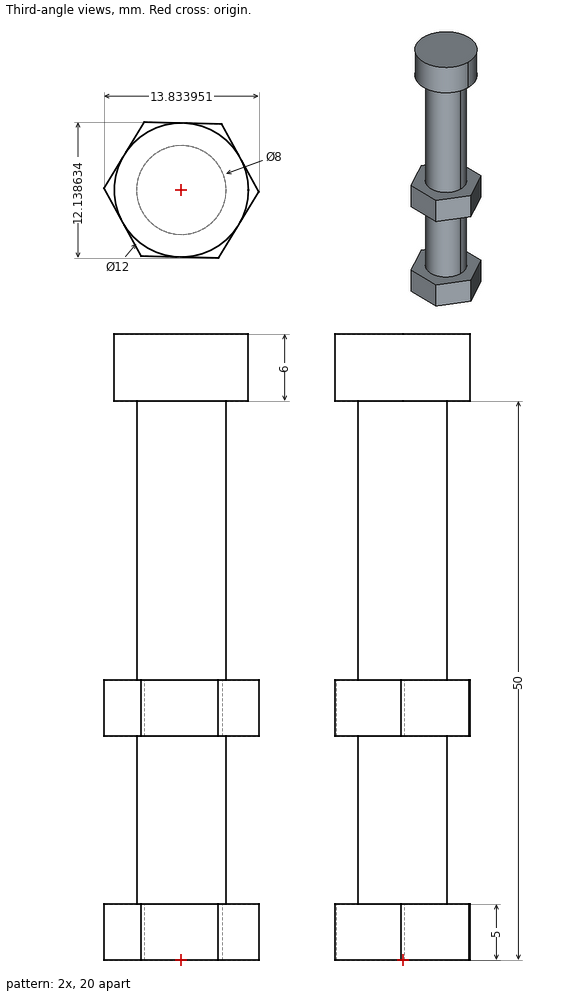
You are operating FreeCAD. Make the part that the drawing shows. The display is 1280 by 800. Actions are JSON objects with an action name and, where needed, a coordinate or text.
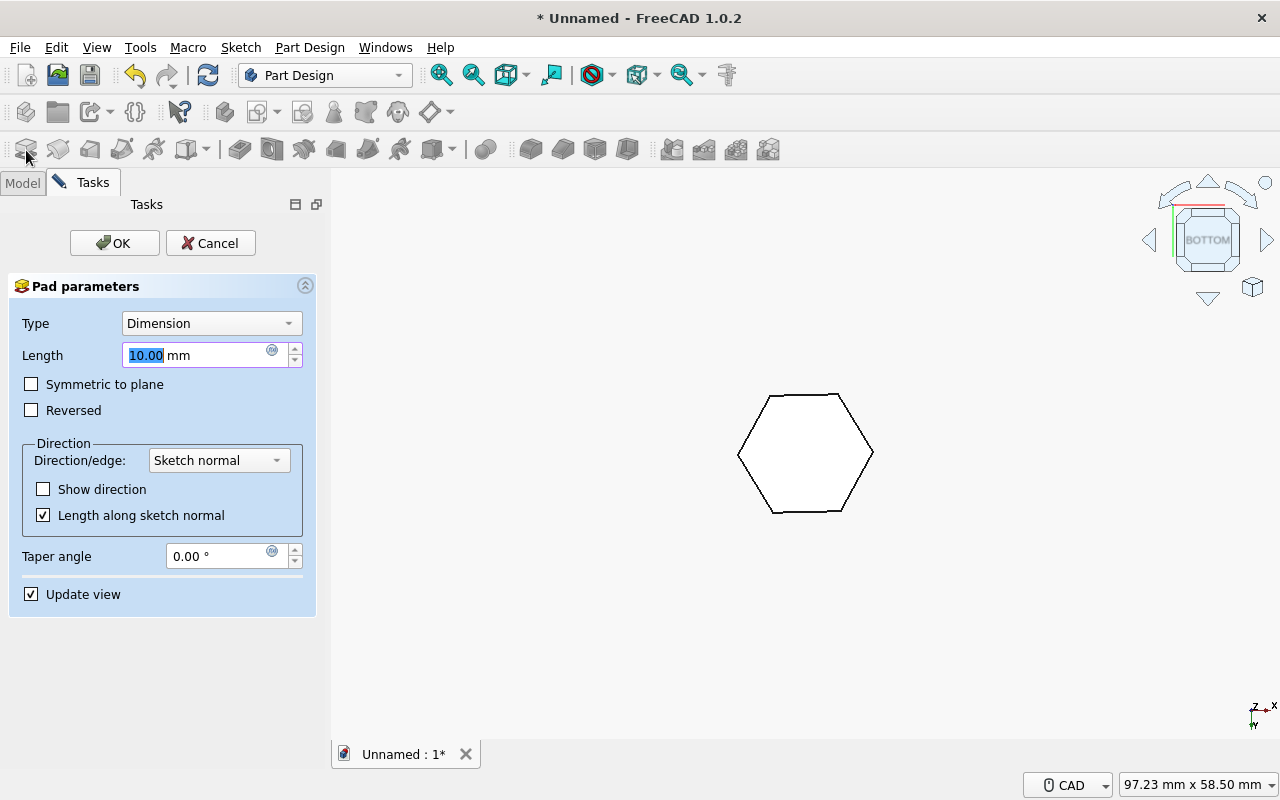
{"action": "type", "text": "5"}
{"action": "key", "text": "Tab"}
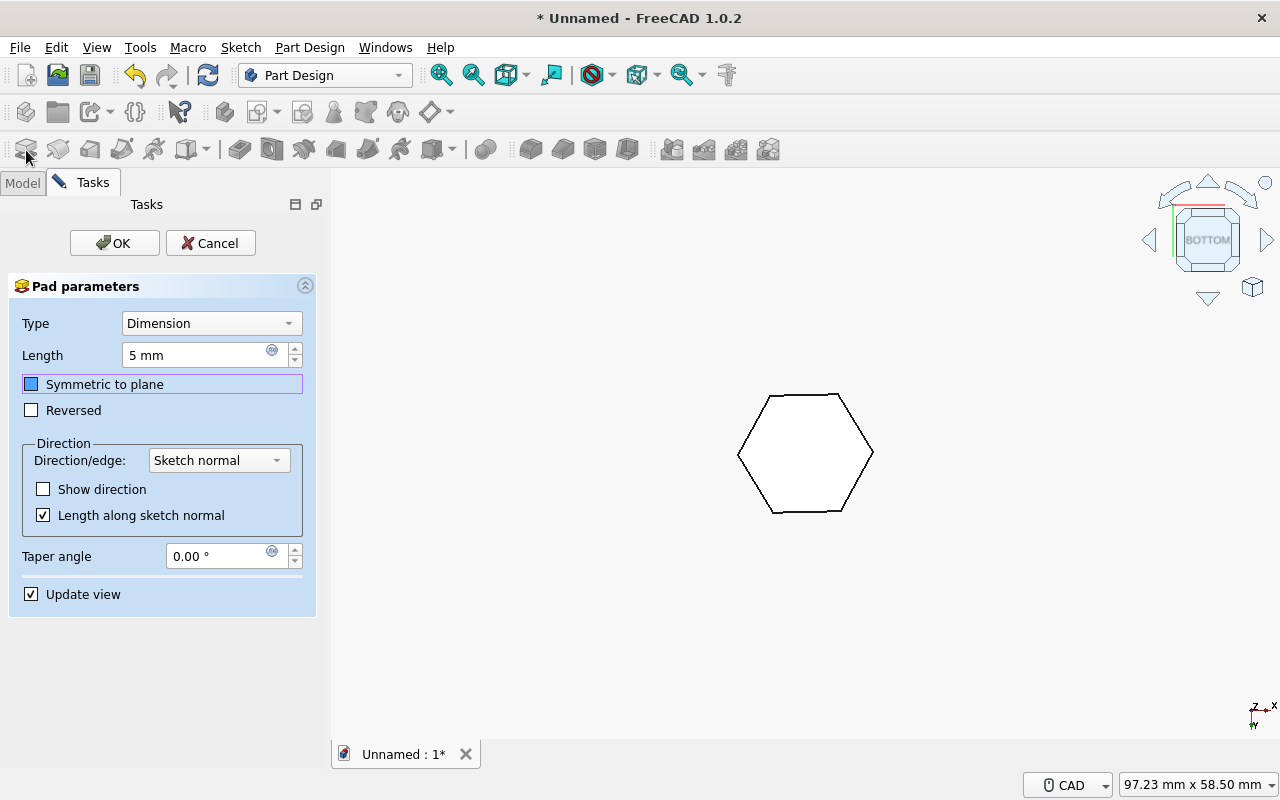
{"action": "left_click", "coordinate": [30, 410]}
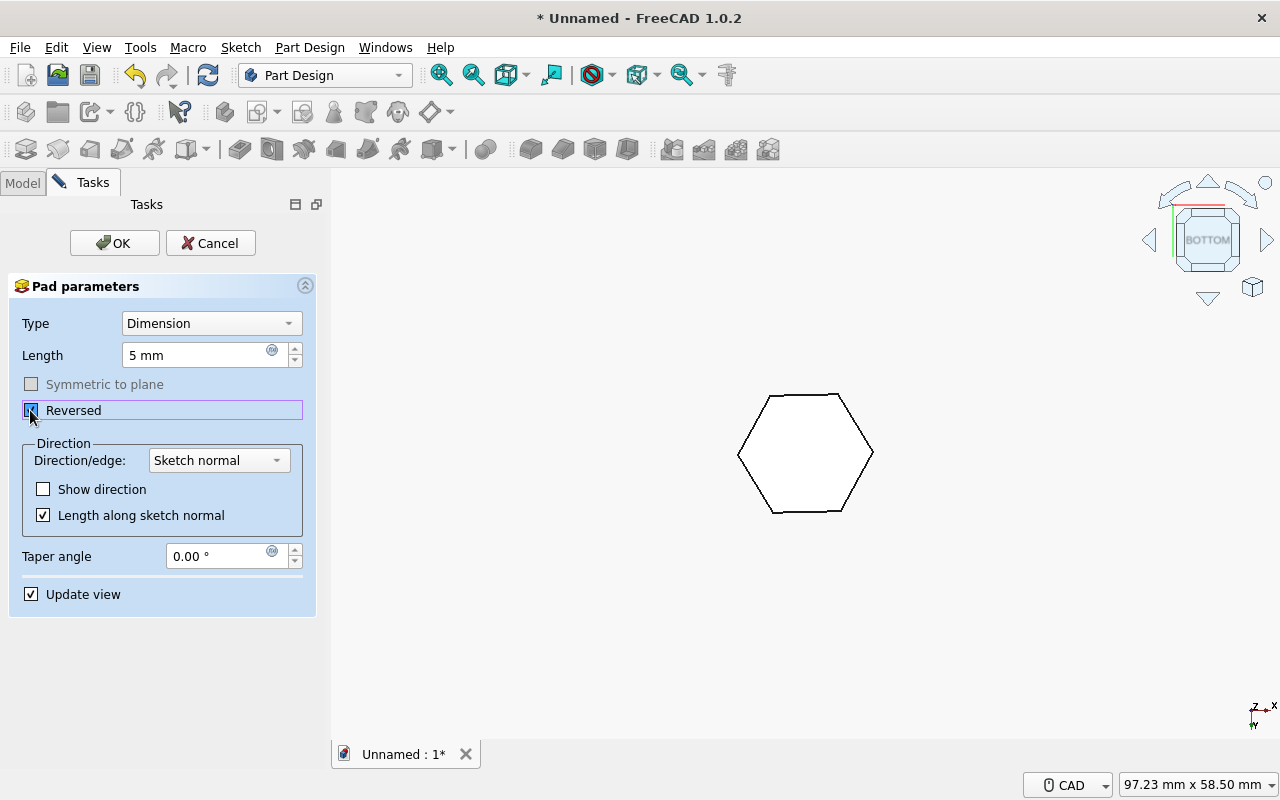
{"action": "left_click", "coordinate": [115, 243]}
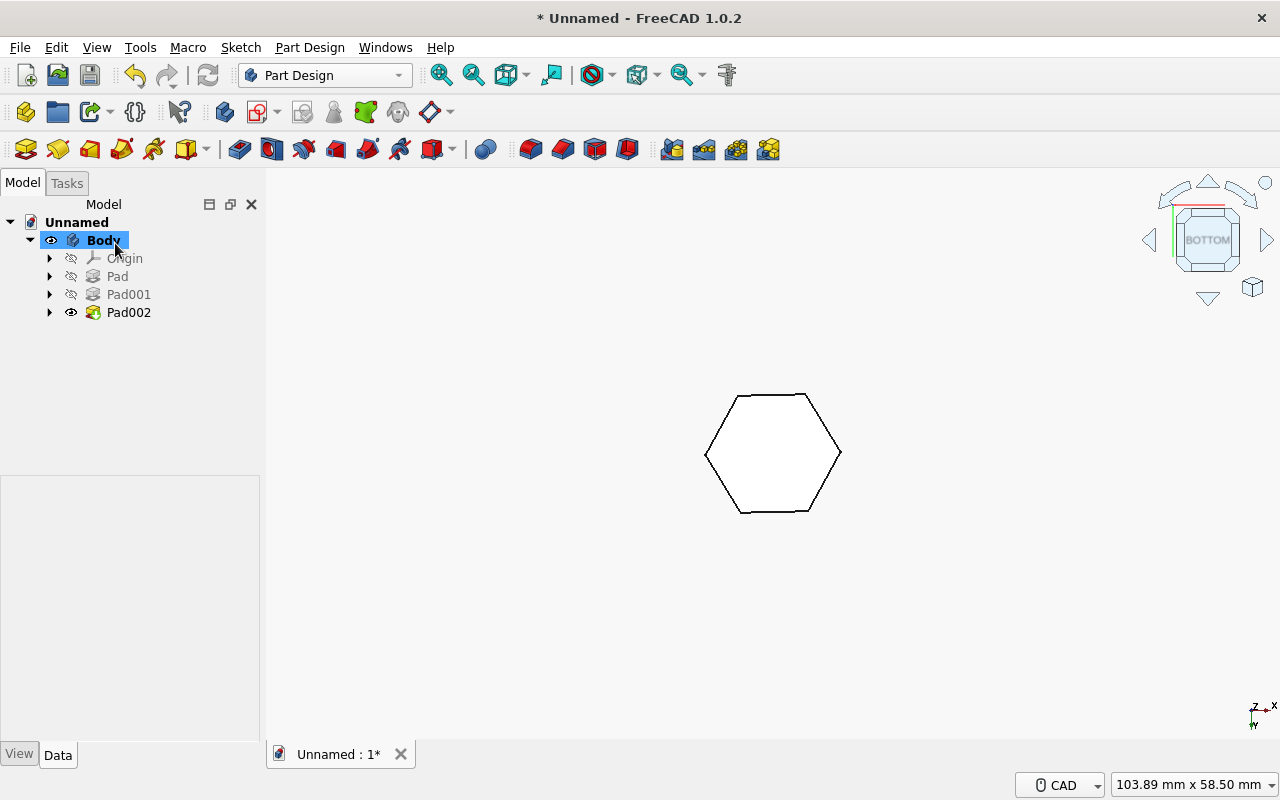
{"action": "left_click", "coordinate": [442, 76]}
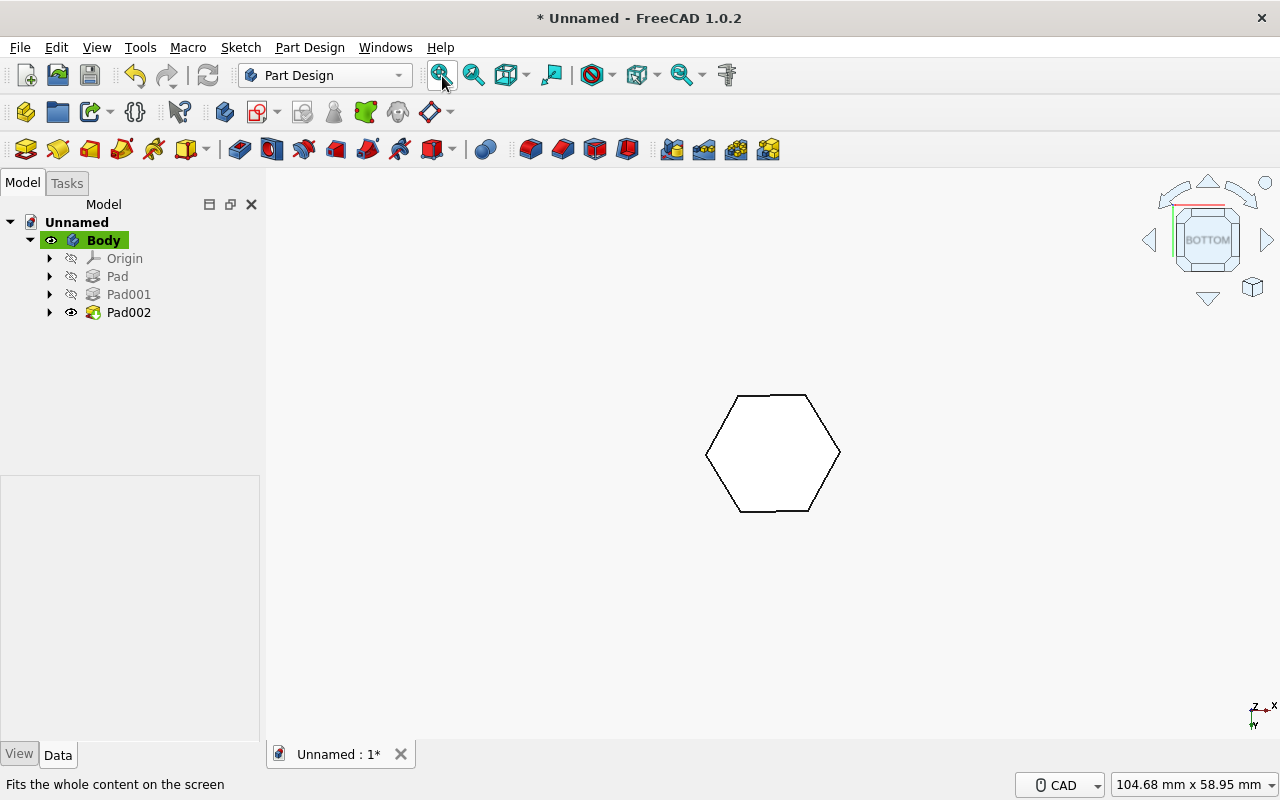
{"action": "left_click", "coordinate": [116, 312]}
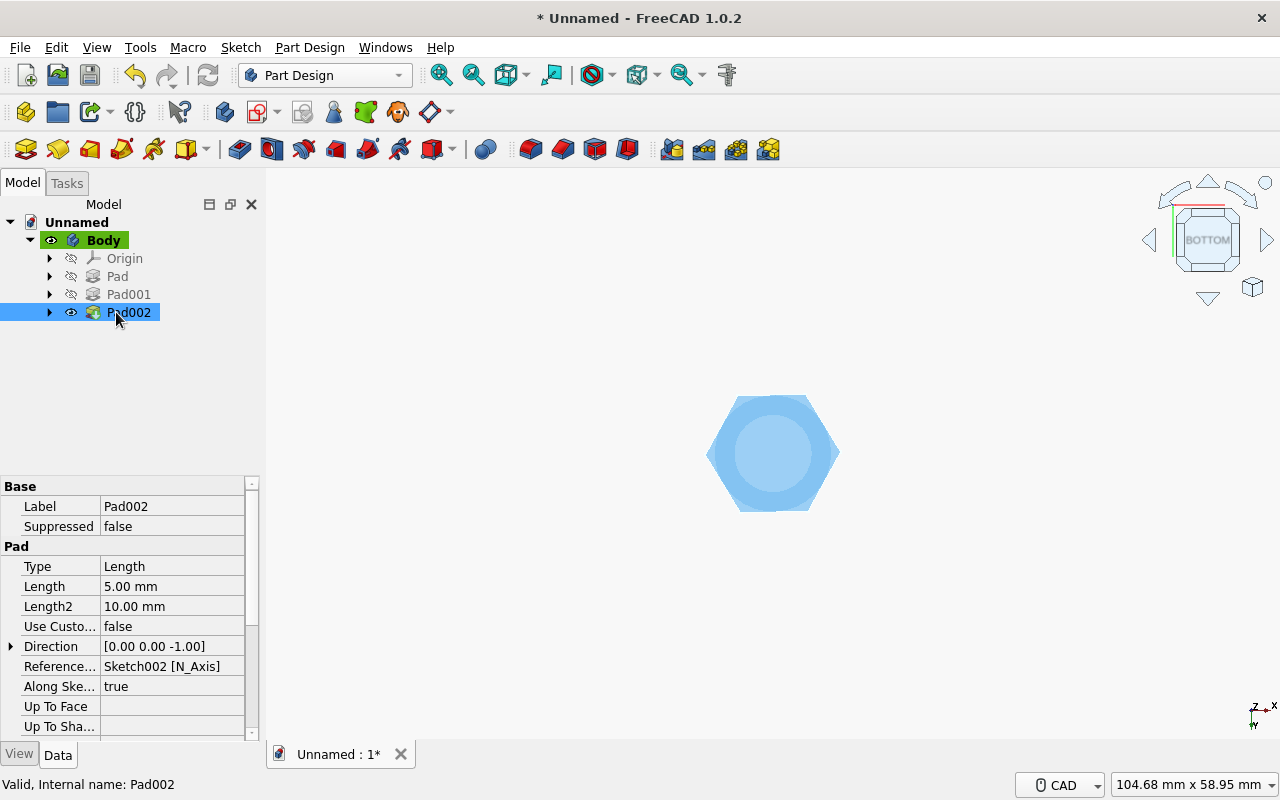
{"action": "left_click", "coordinate": [704, 150]}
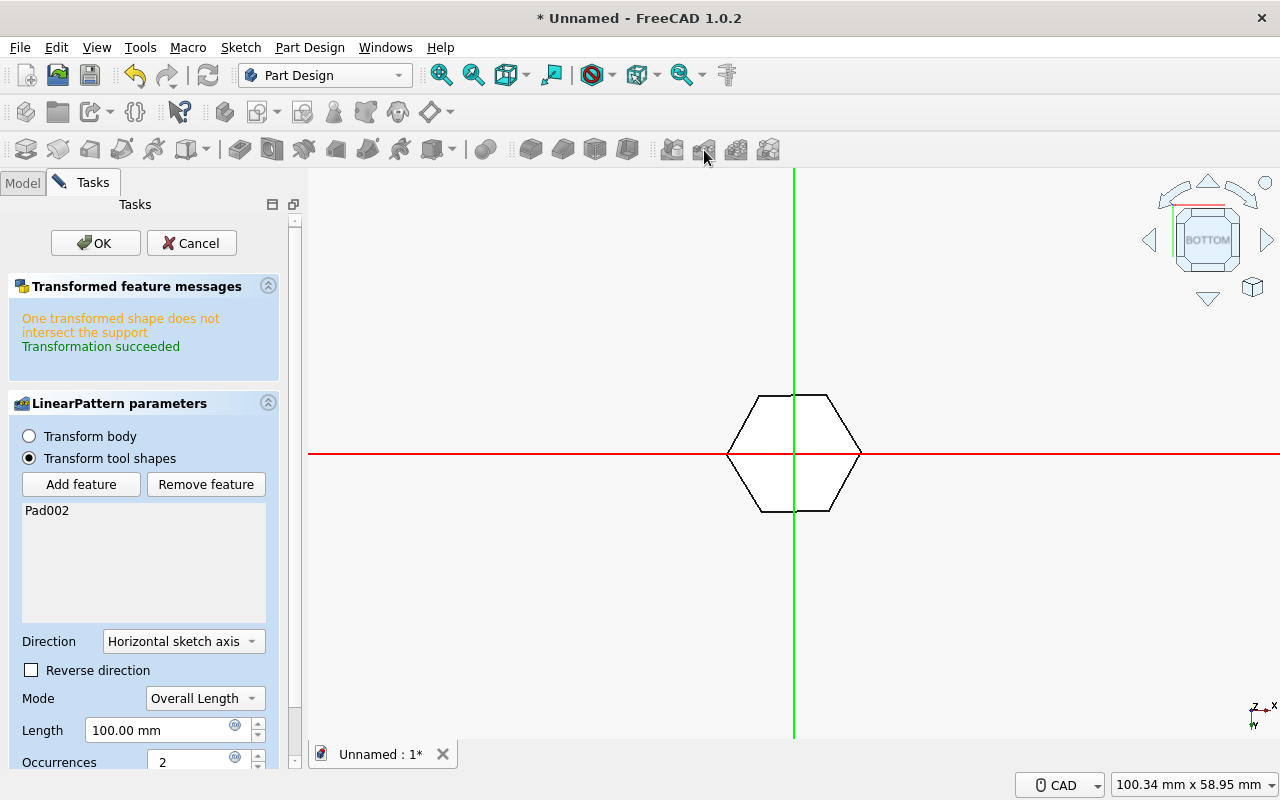
{"action": "left_click", "coordinate": [184, 642]}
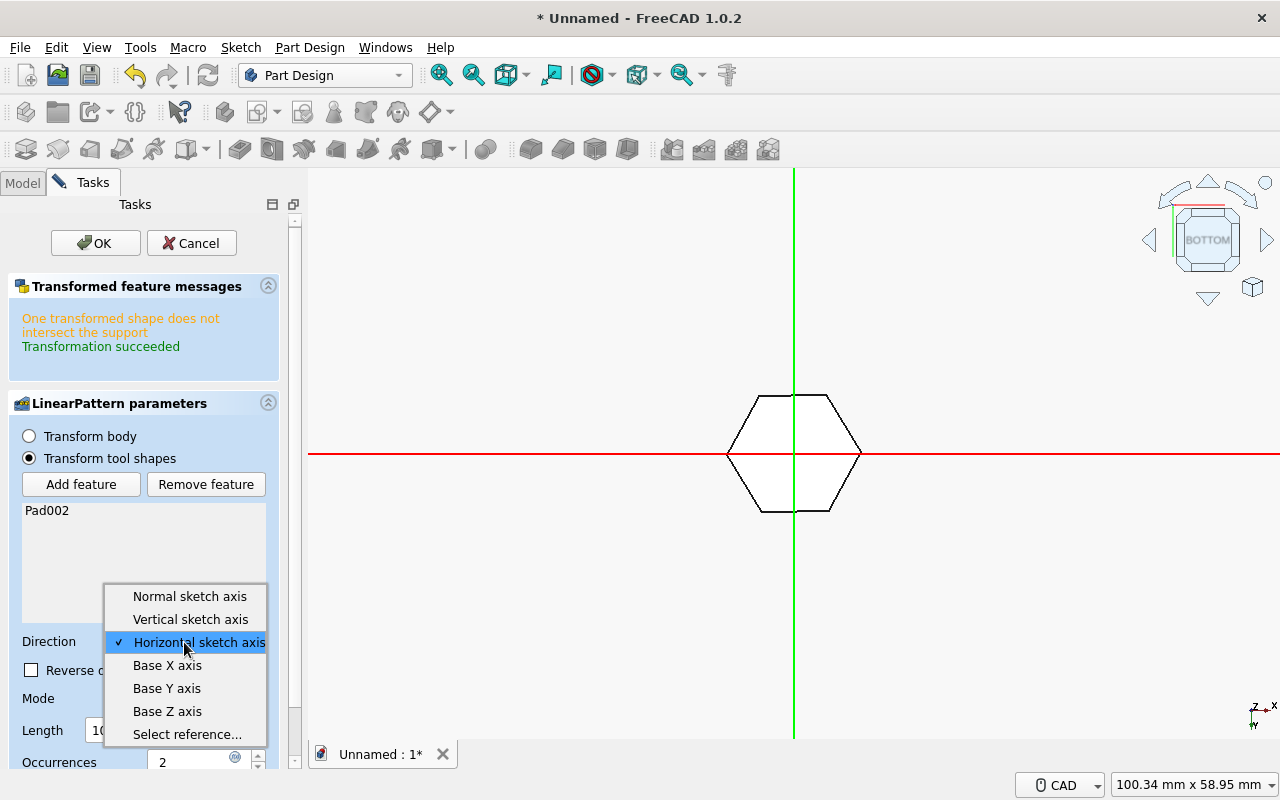
{"action": "left_click", "coordinate": [184, 712]}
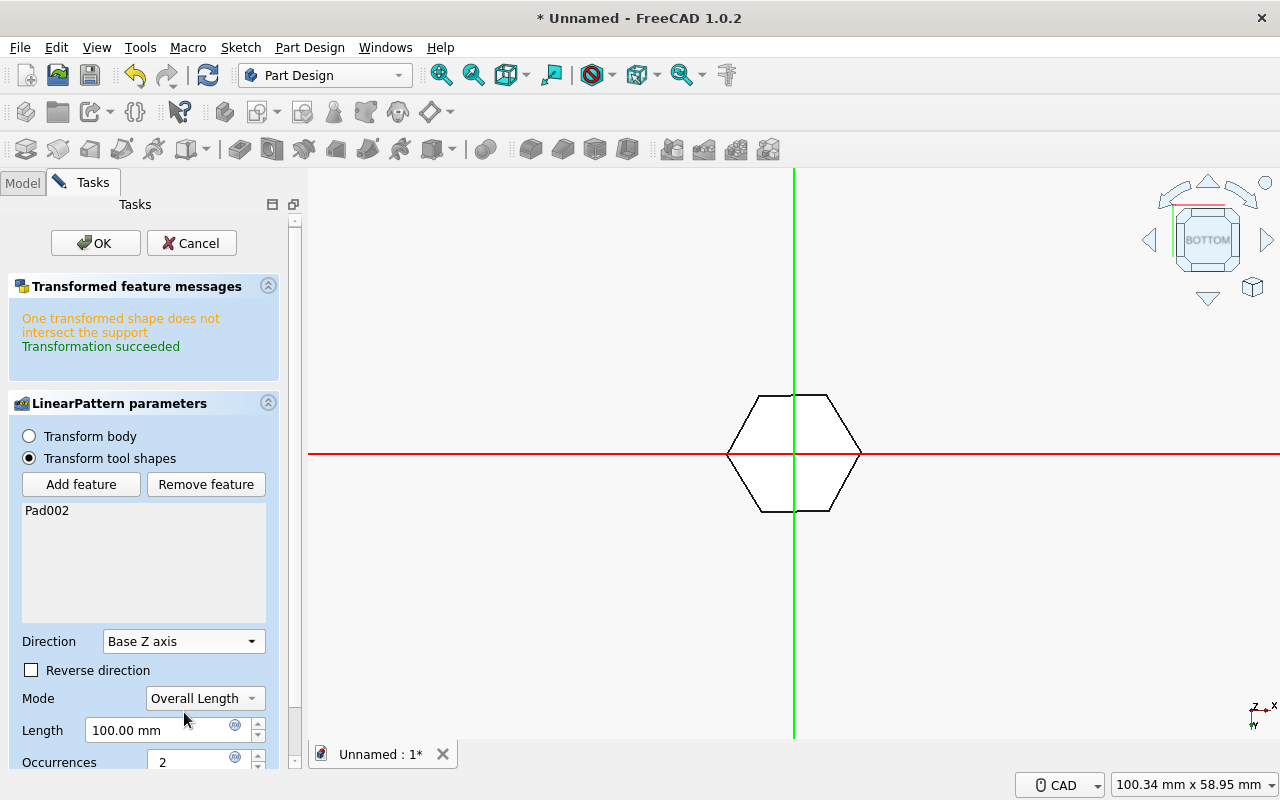
{"action": "left_click", "coordinate": [206, 698]}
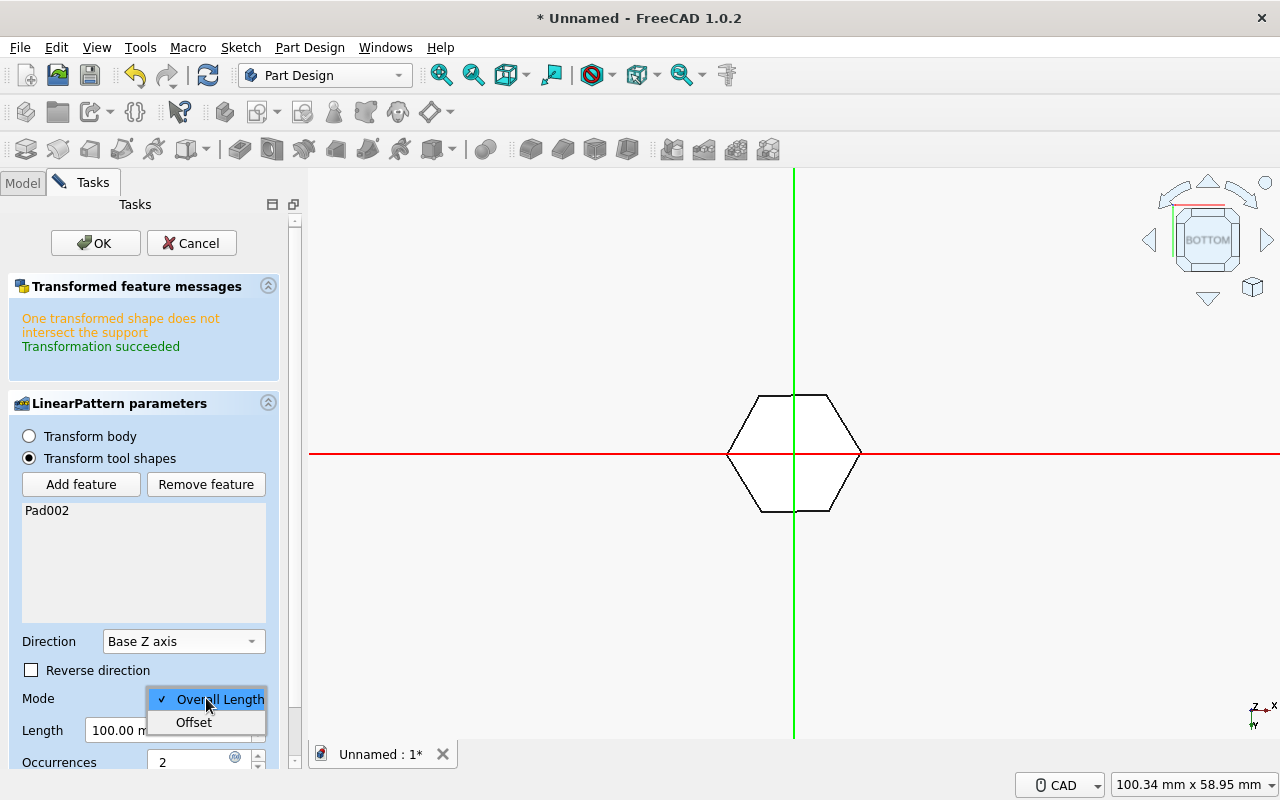
{"action": "left_click", "coordinate": [206, 722]}